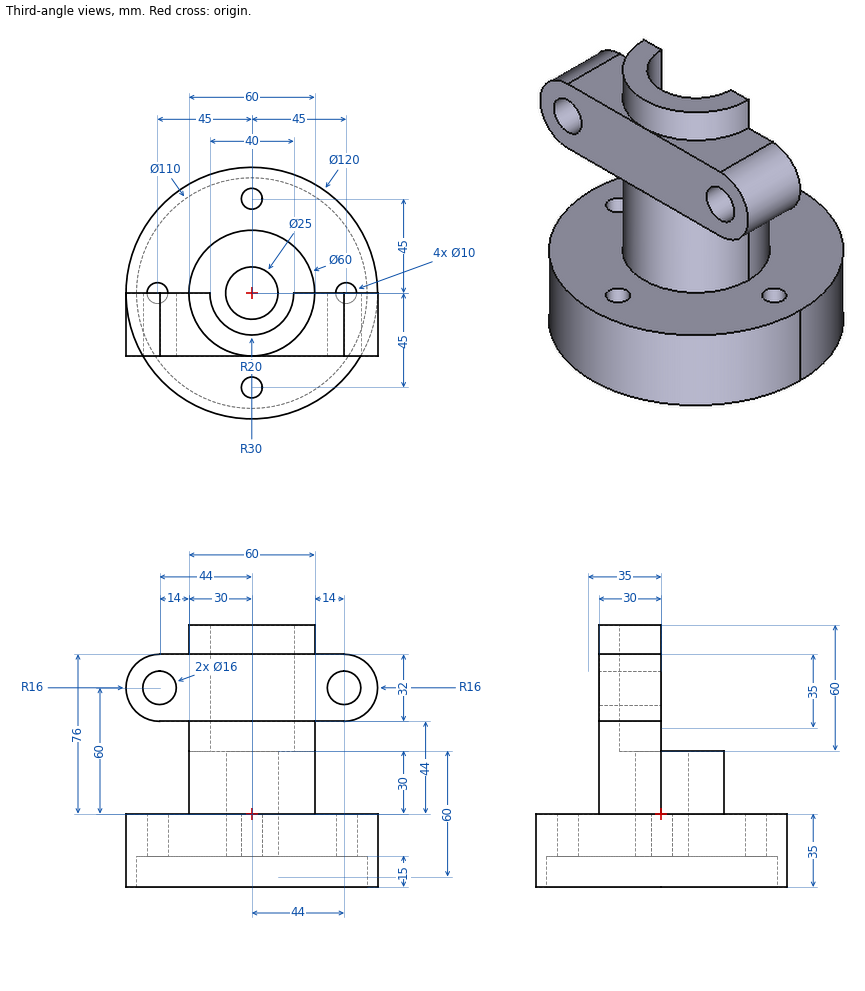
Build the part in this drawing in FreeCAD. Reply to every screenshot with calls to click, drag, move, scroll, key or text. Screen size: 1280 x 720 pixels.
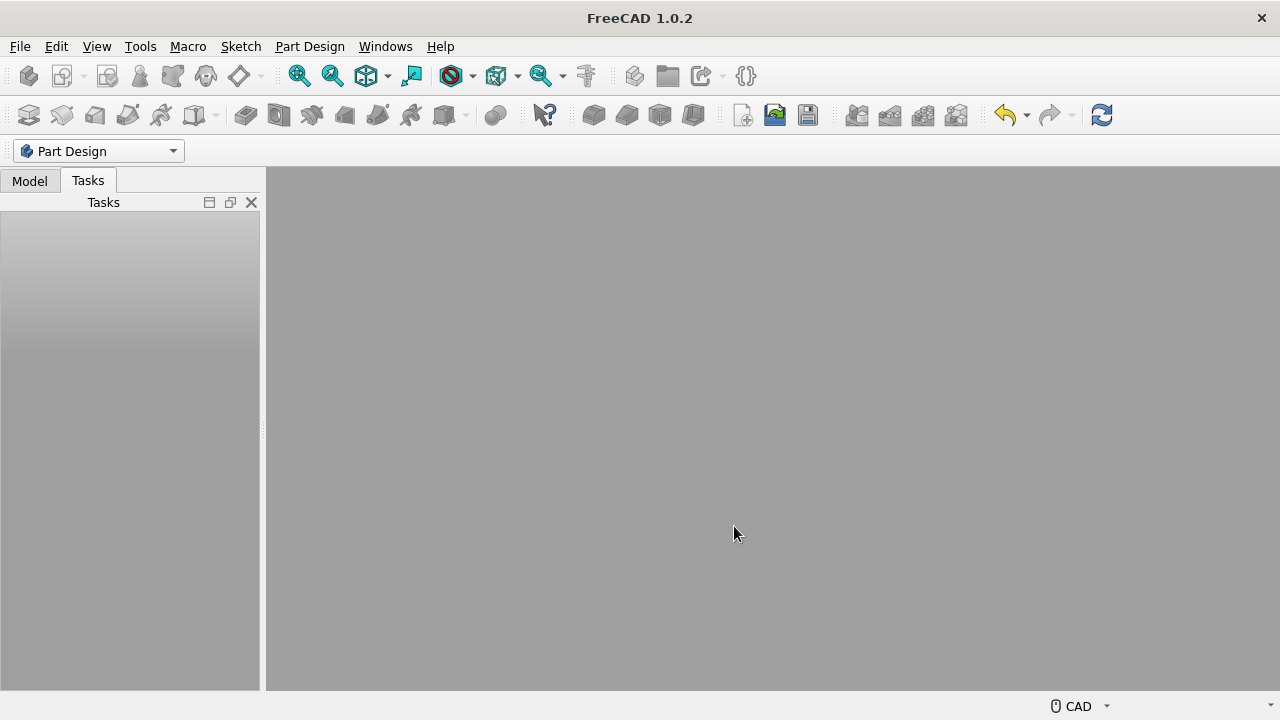
click(742, 116)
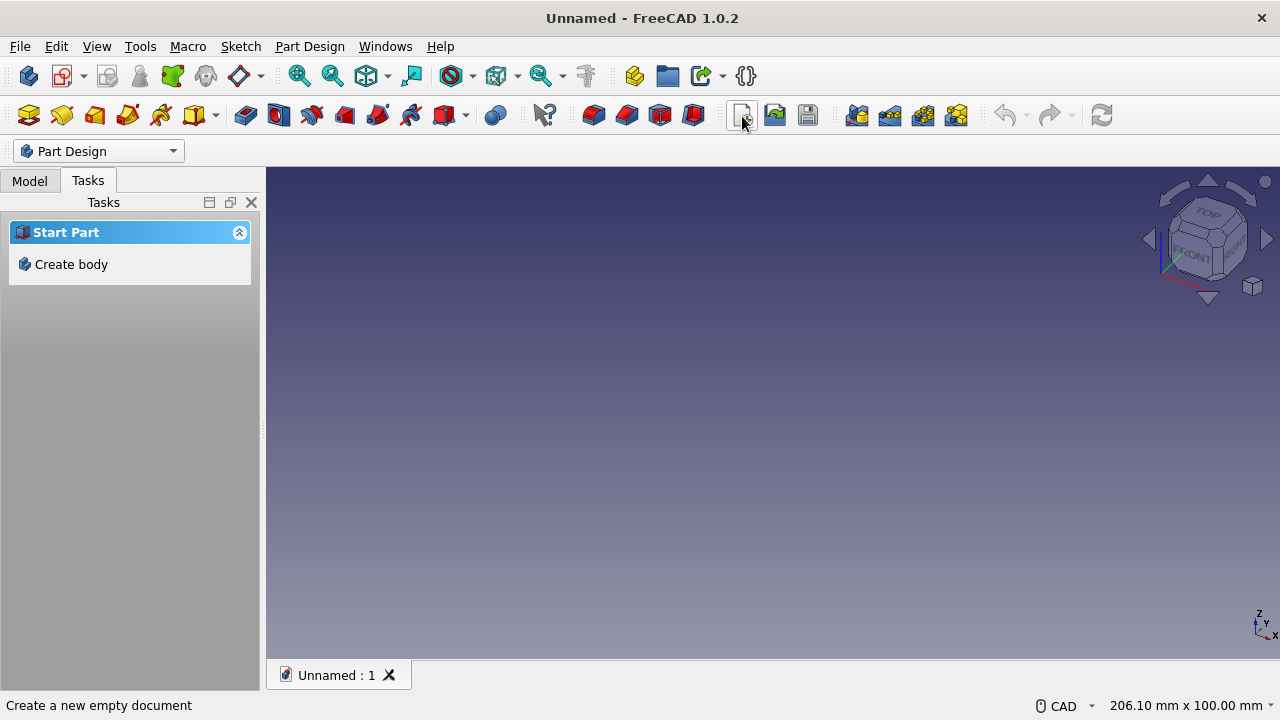
click(62, 76)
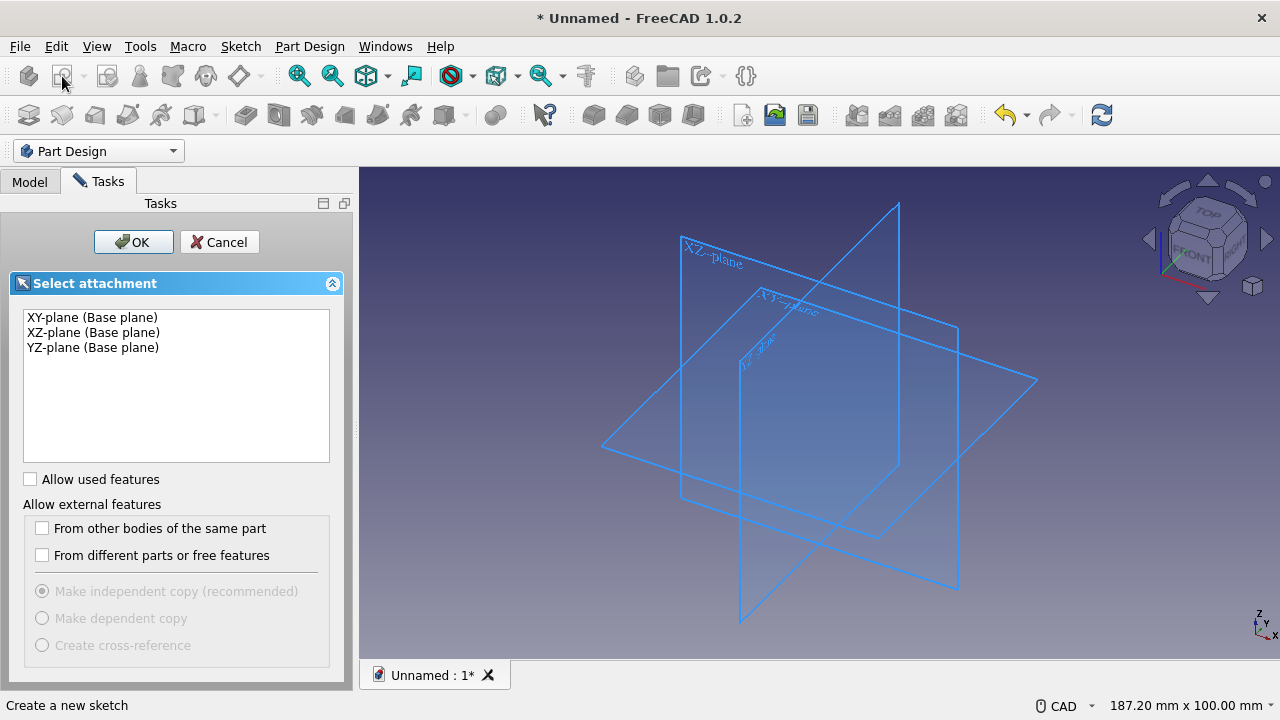
click(84, 318)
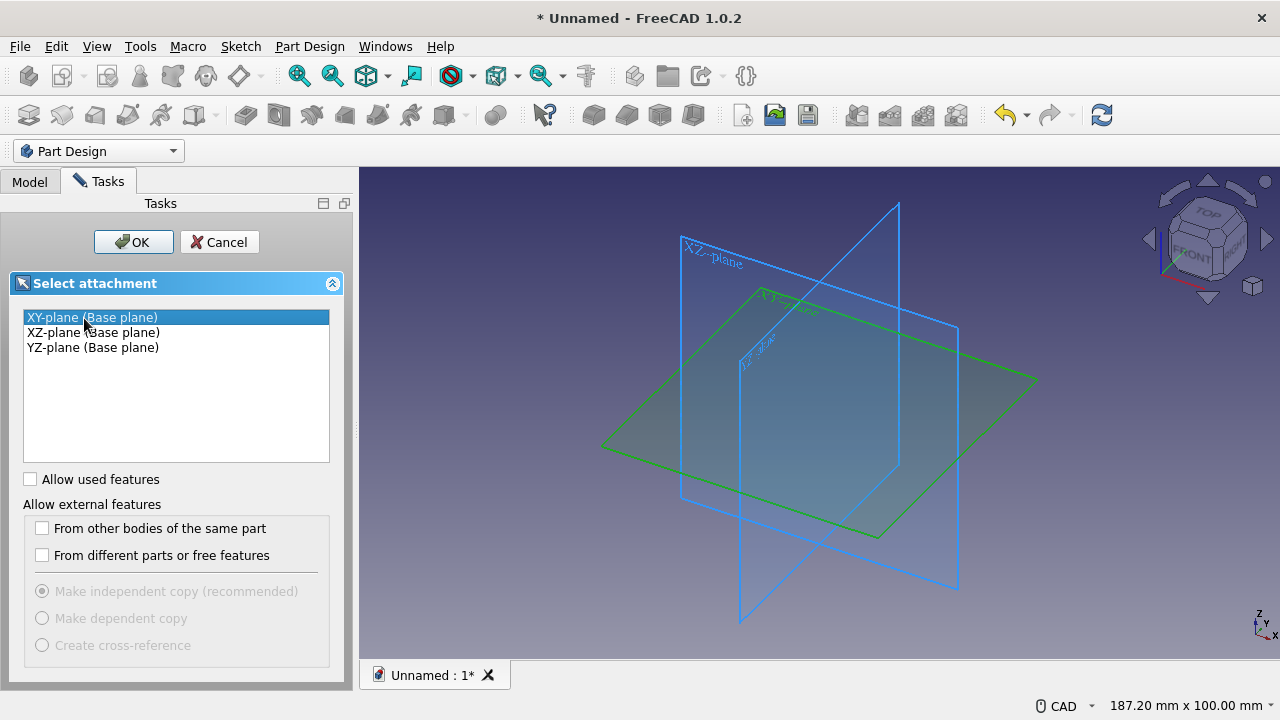
click(134, 242)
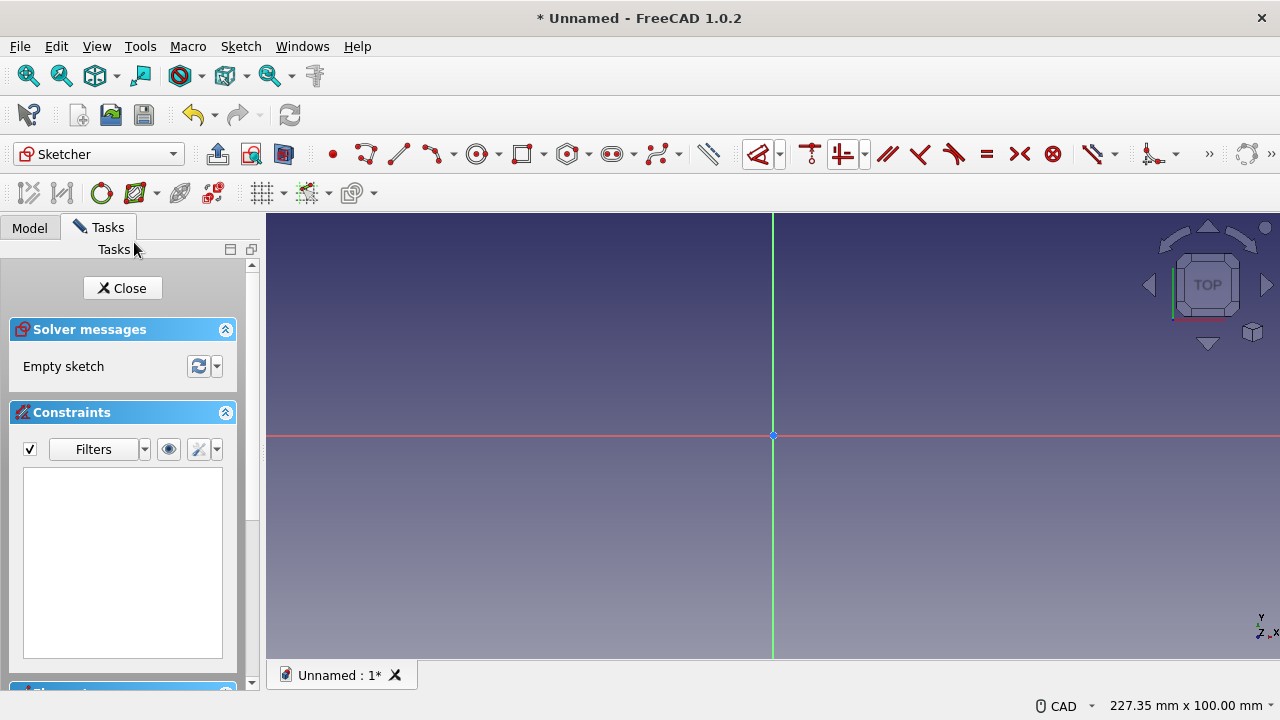
scroll(621, 436, down, 3)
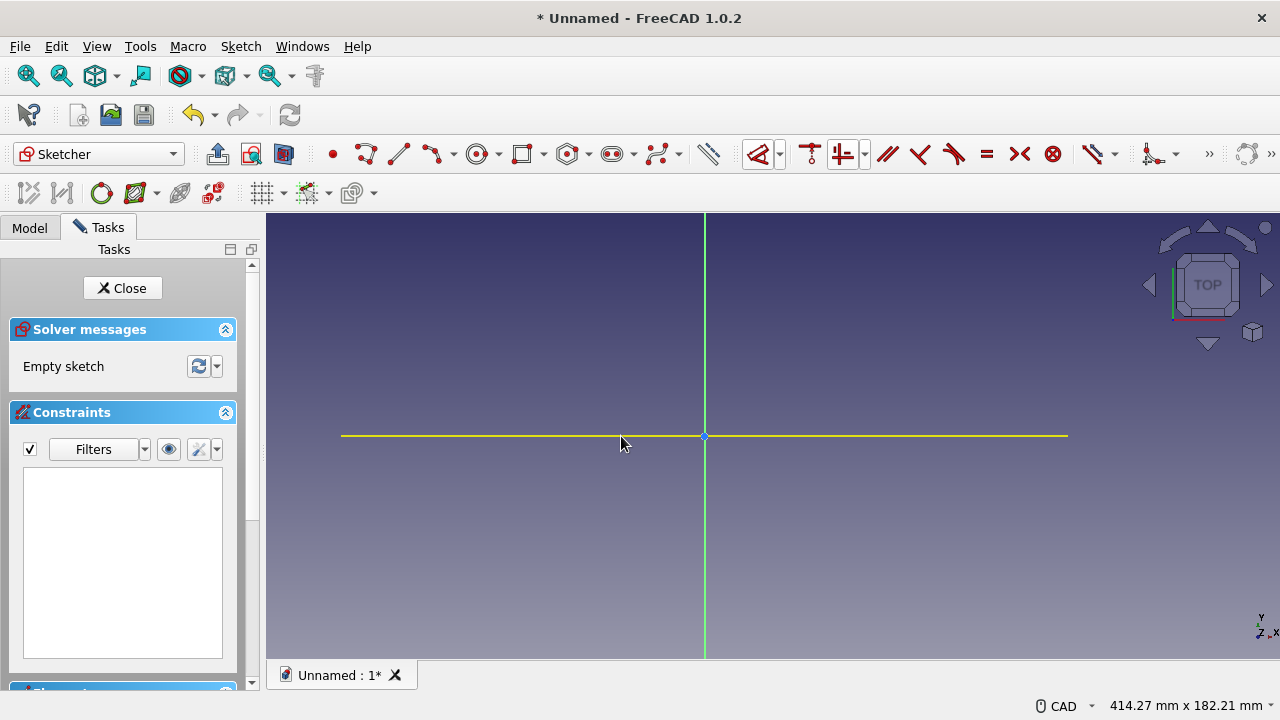
click(476, 154)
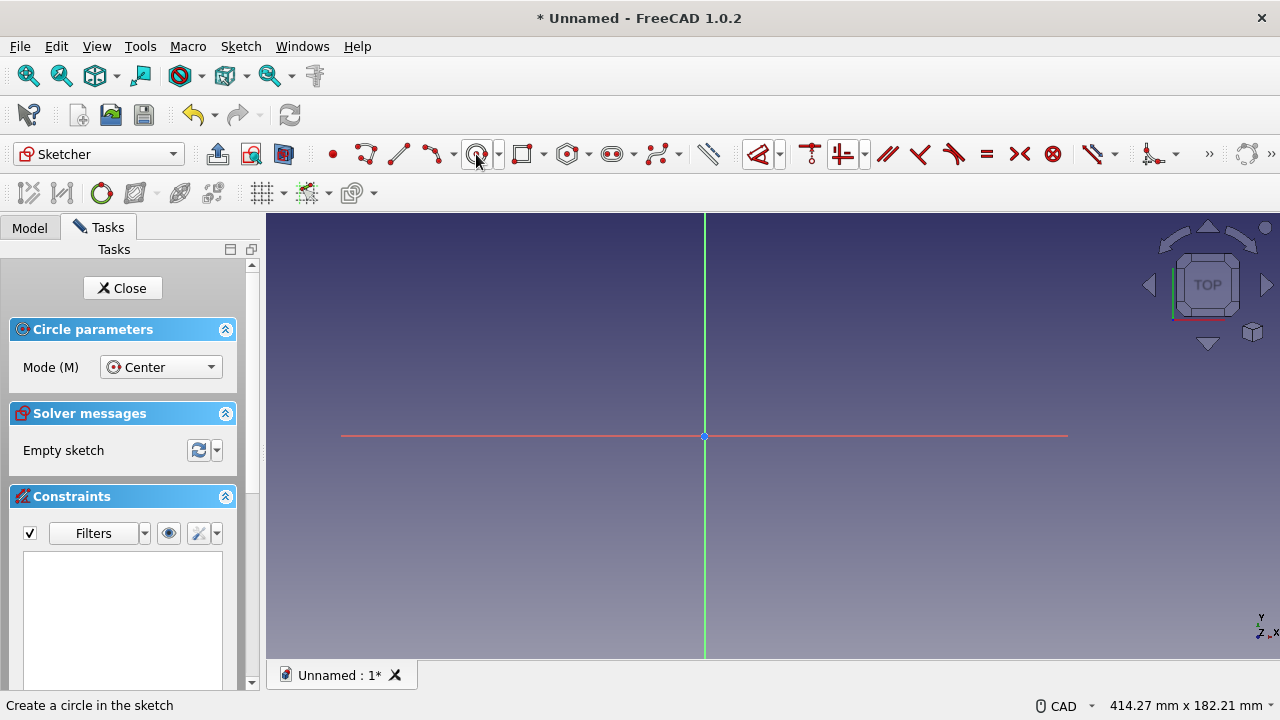
click(705, 436)
move(808, 332)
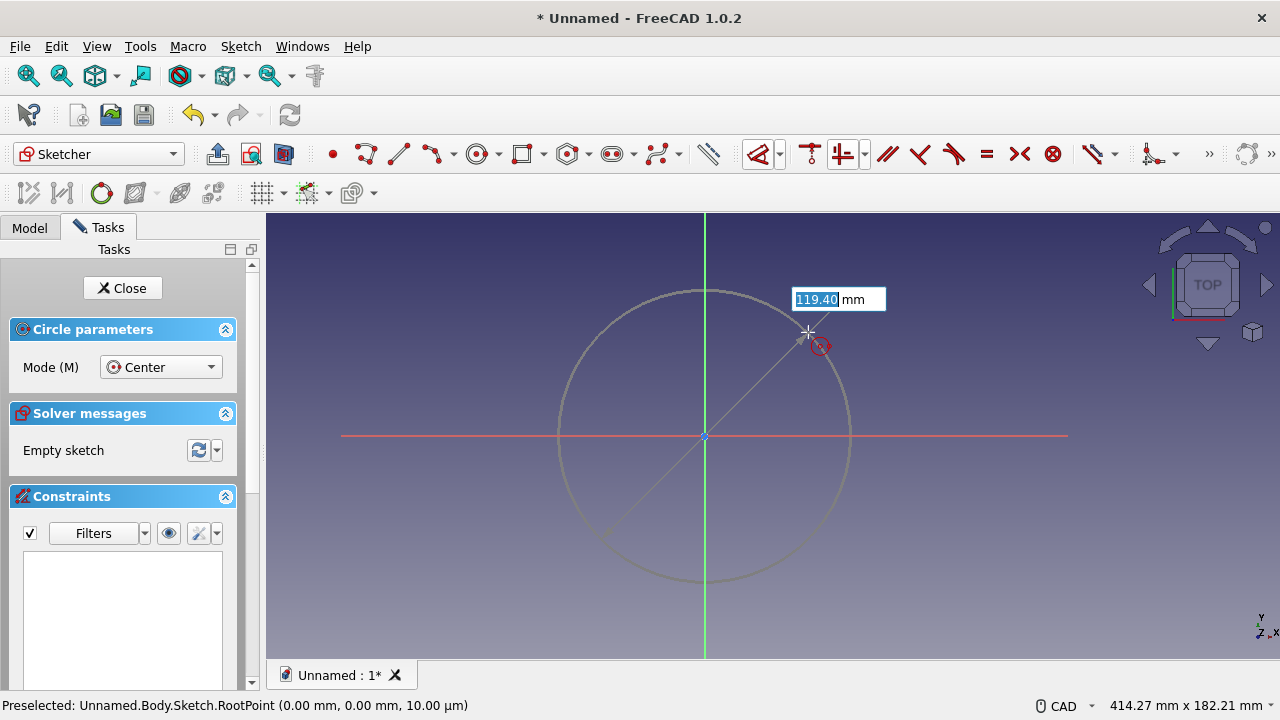
text(120)
key(Return)
key(Escape)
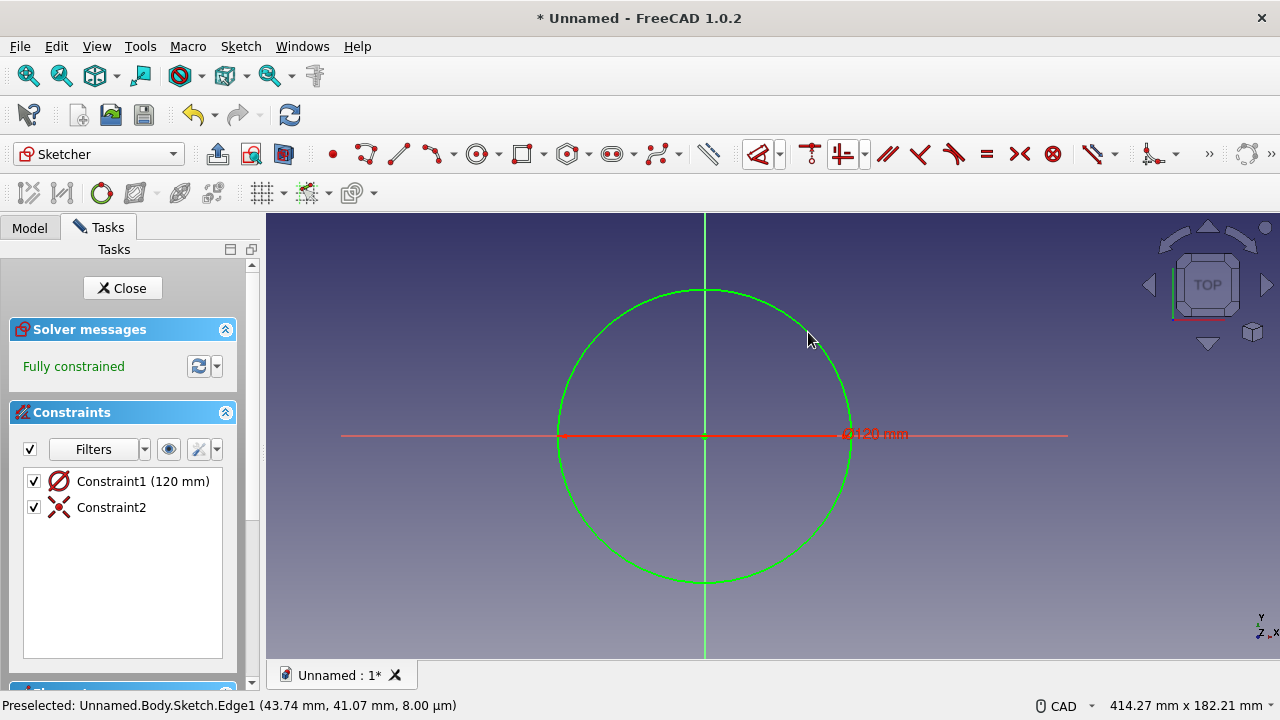
click(123, 288)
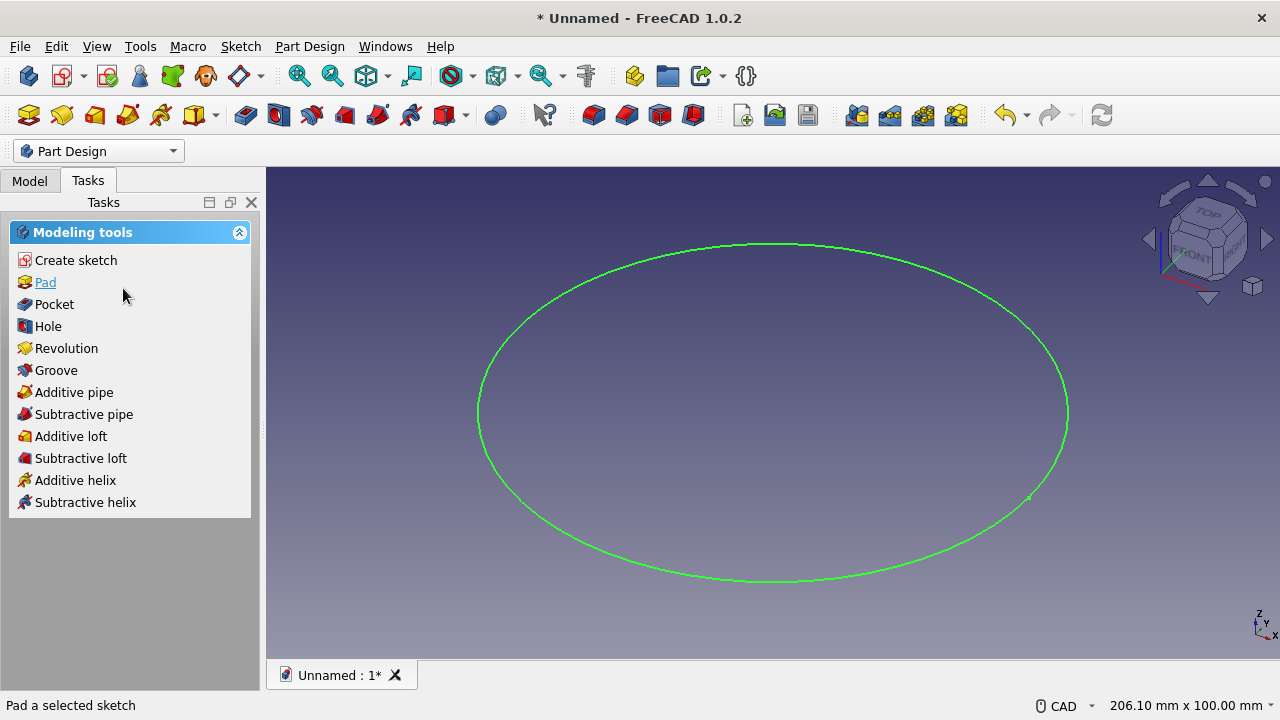
click(29, 116)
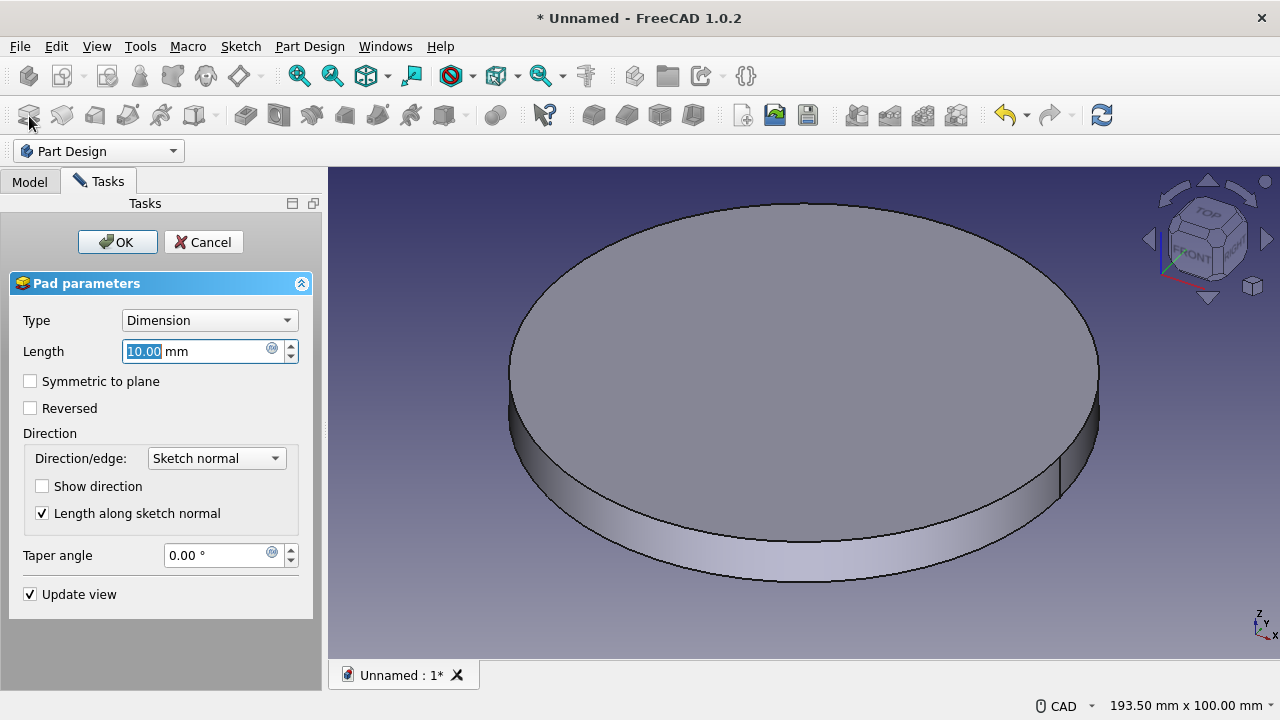
text(35)
key(Tab)